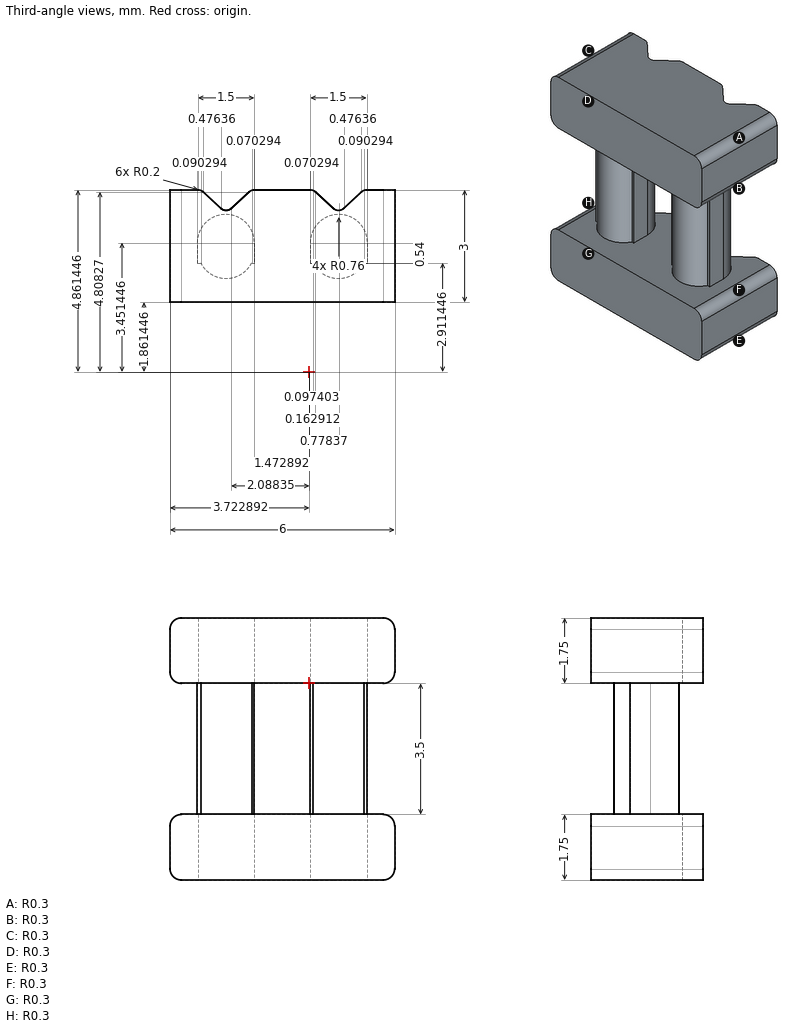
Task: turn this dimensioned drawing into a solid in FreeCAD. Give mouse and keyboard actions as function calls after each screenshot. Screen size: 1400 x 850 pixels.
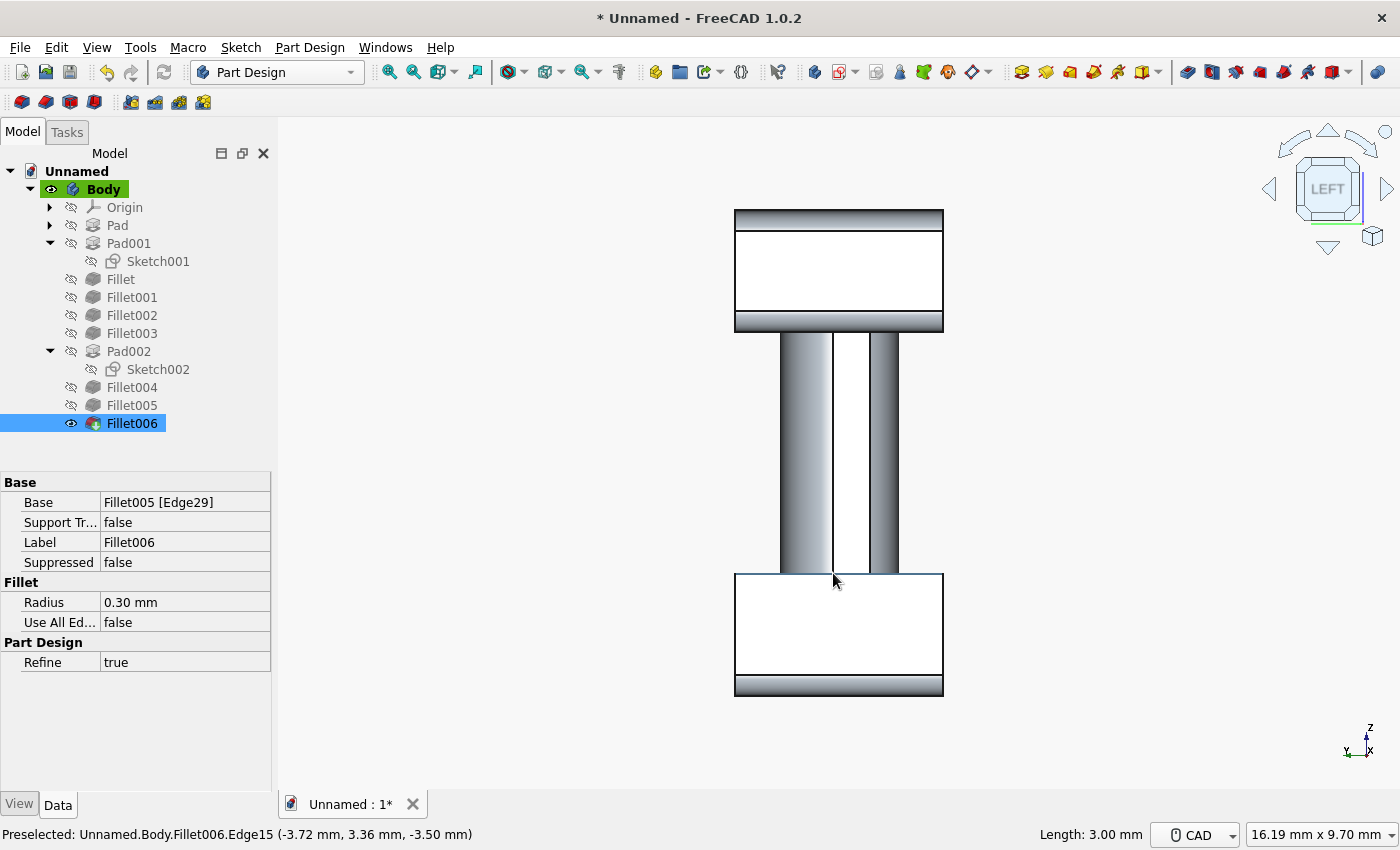
click(22, 102)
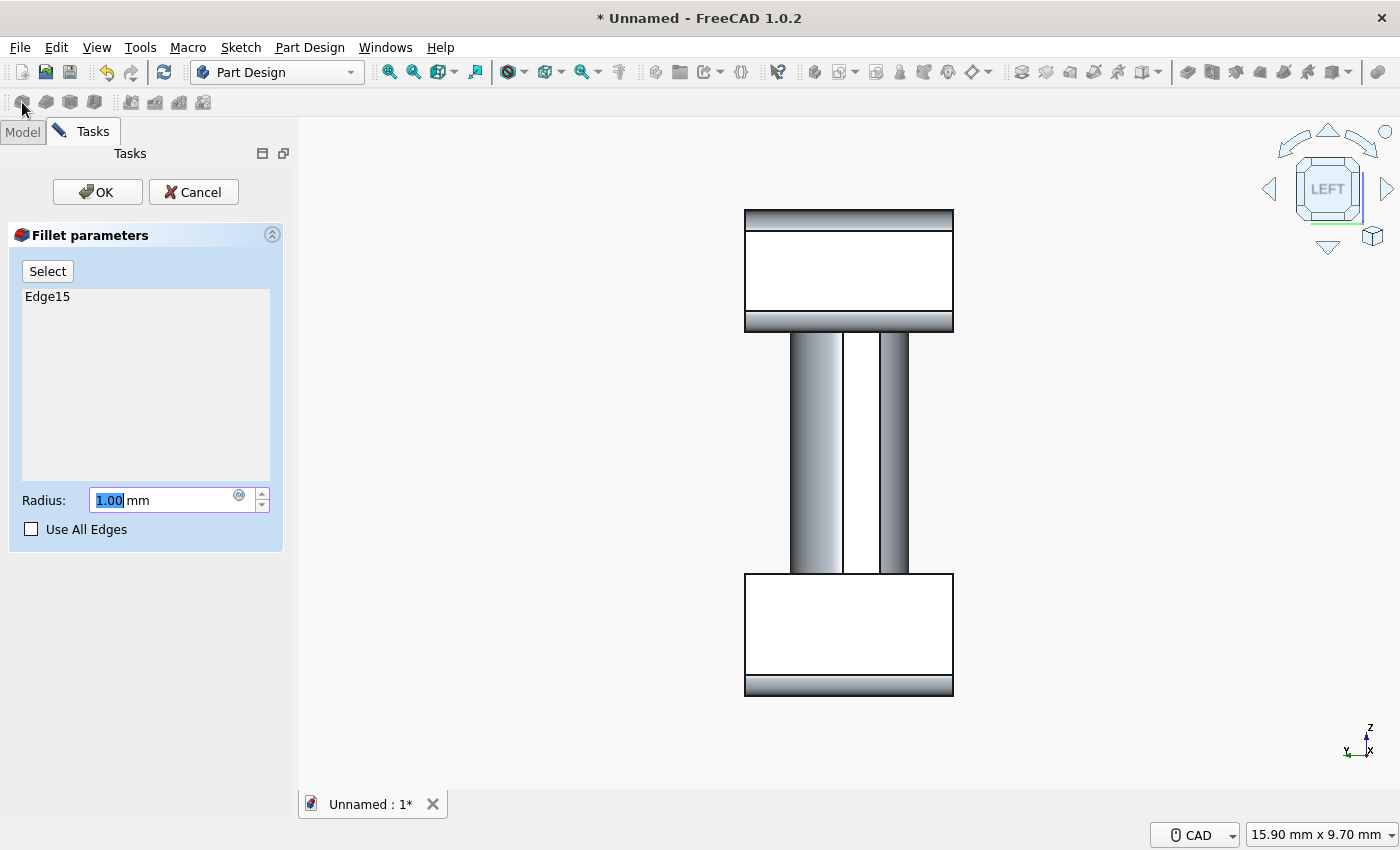
text(0.3)
key(Tab)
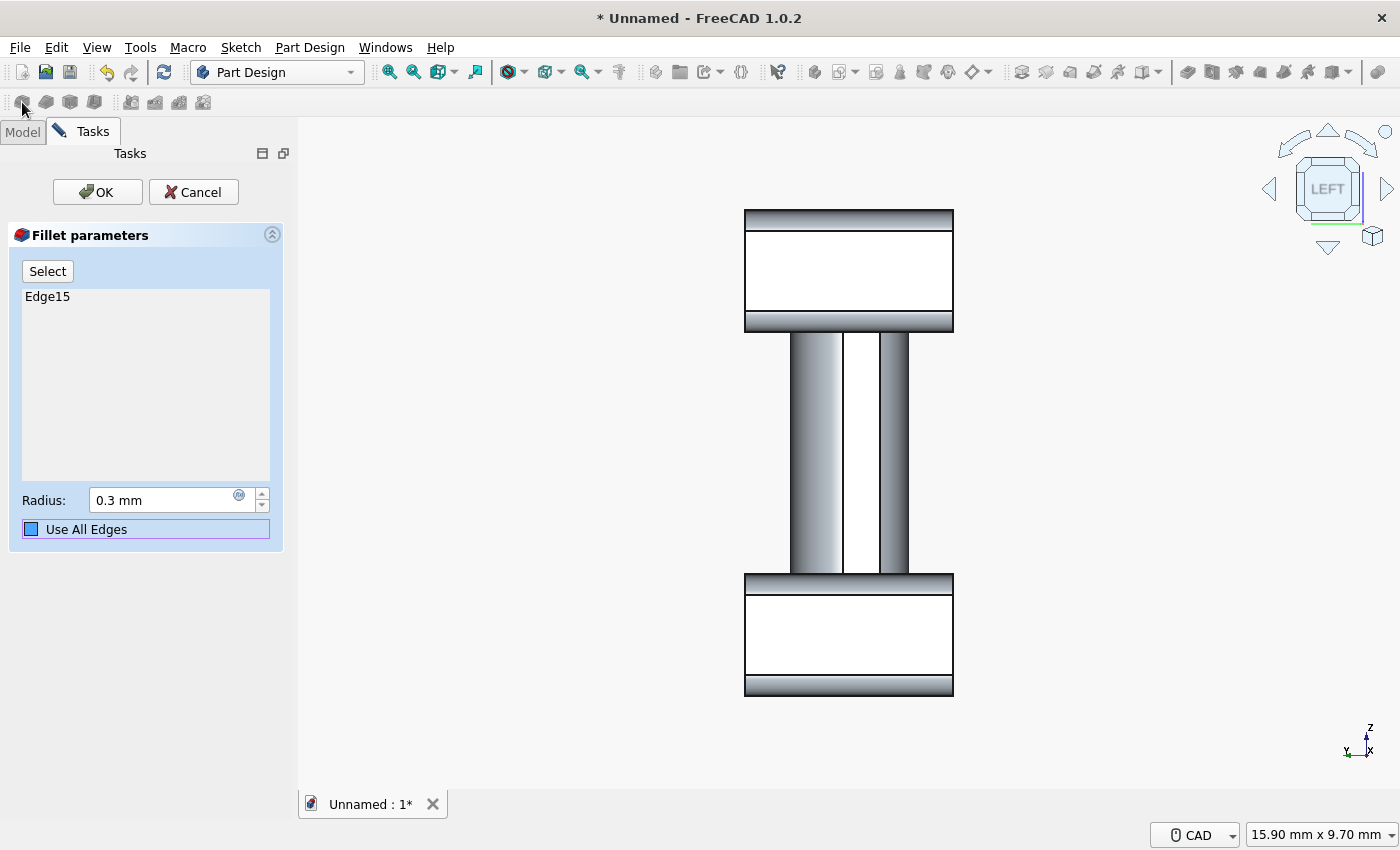
click(98, 192)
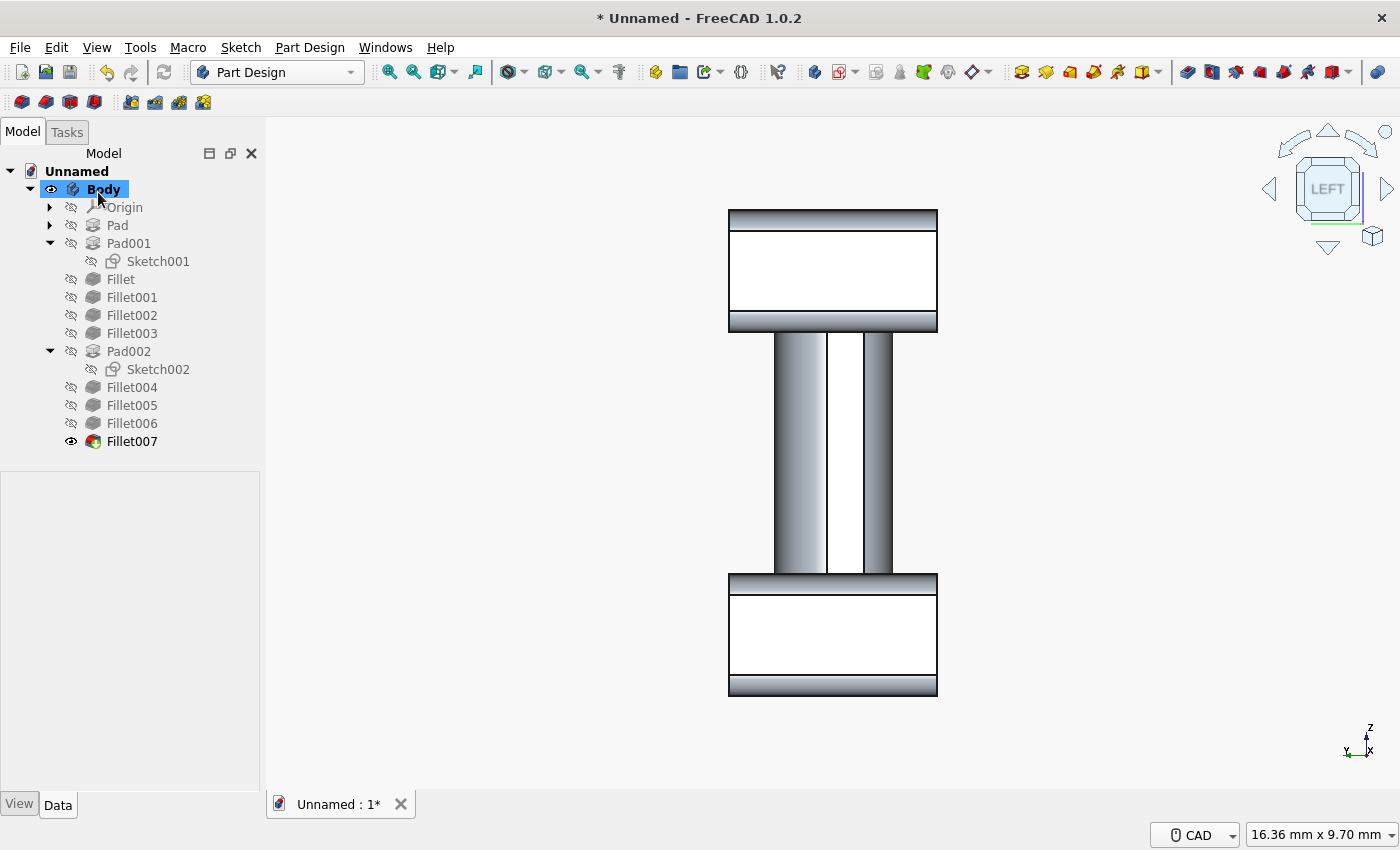
key(0)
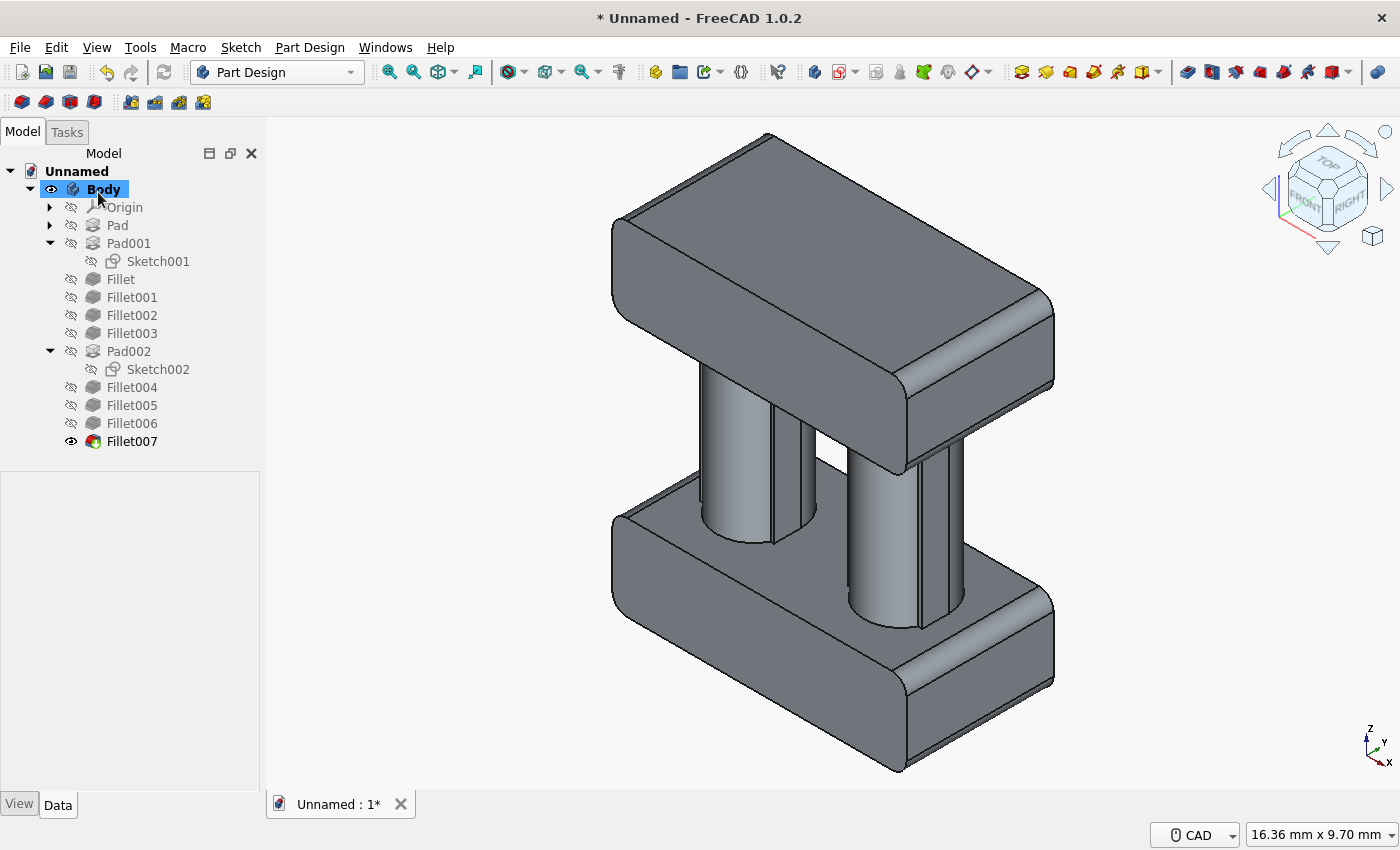
click(871, 276)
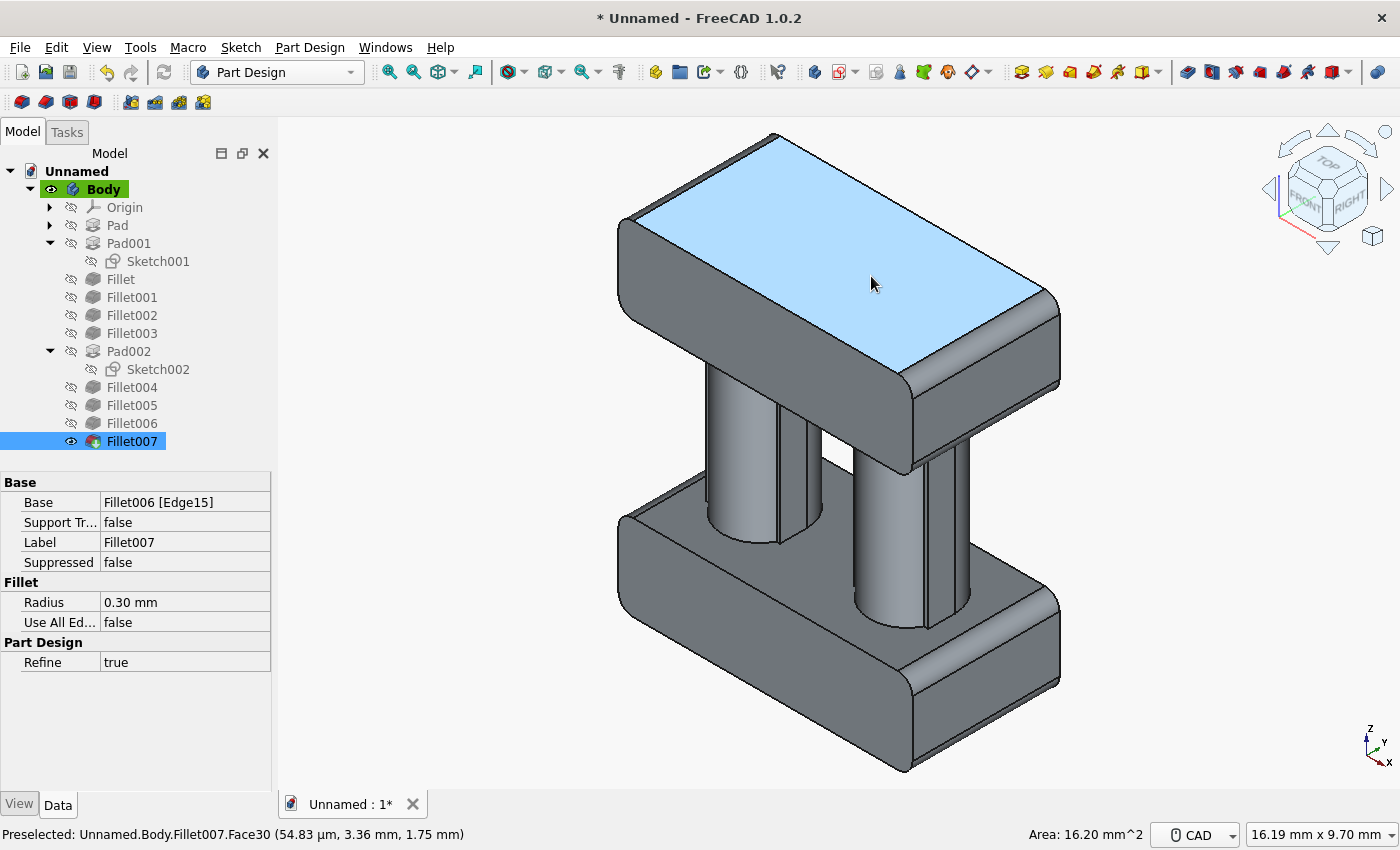
click(840, 72)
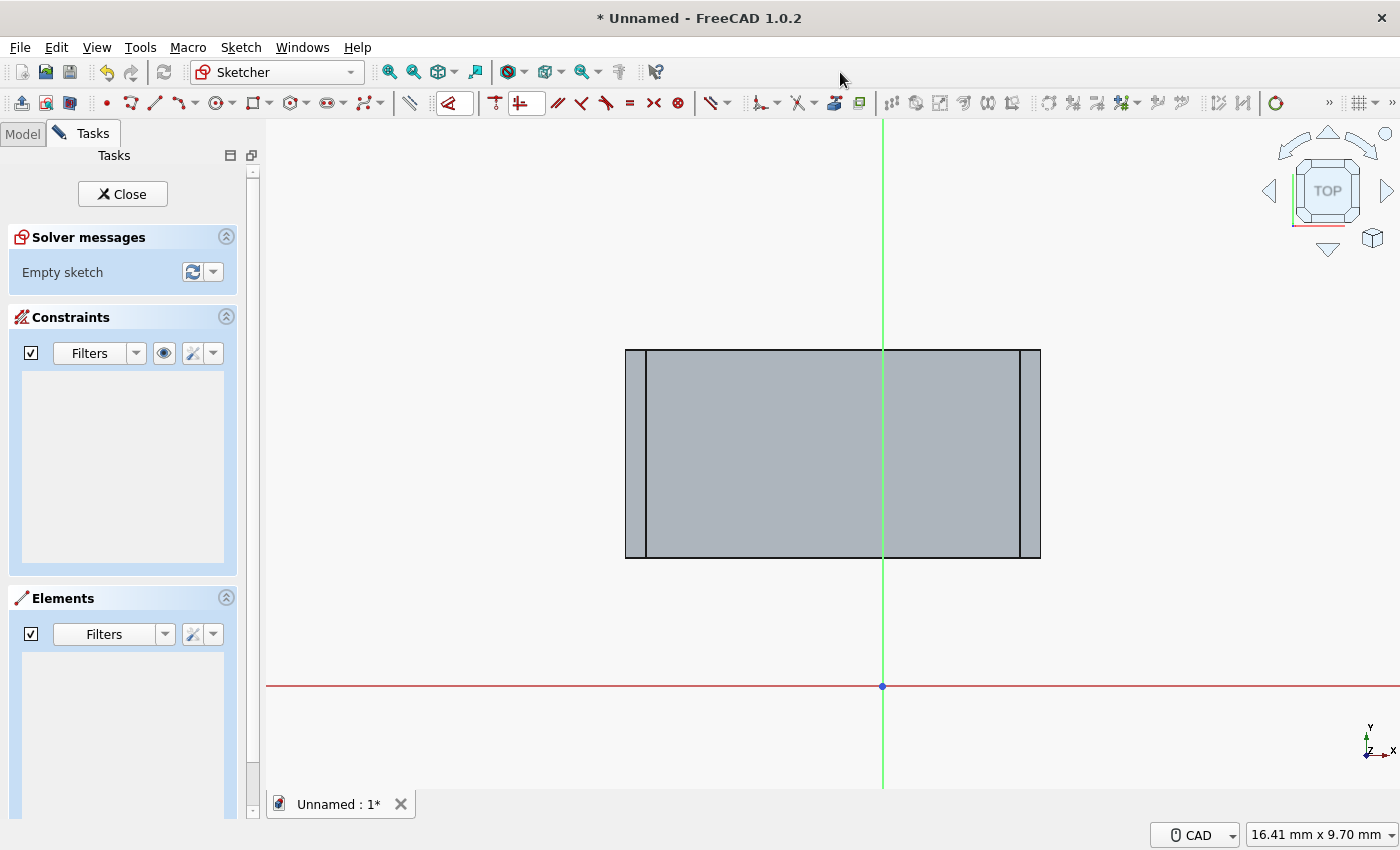
click(156, 104)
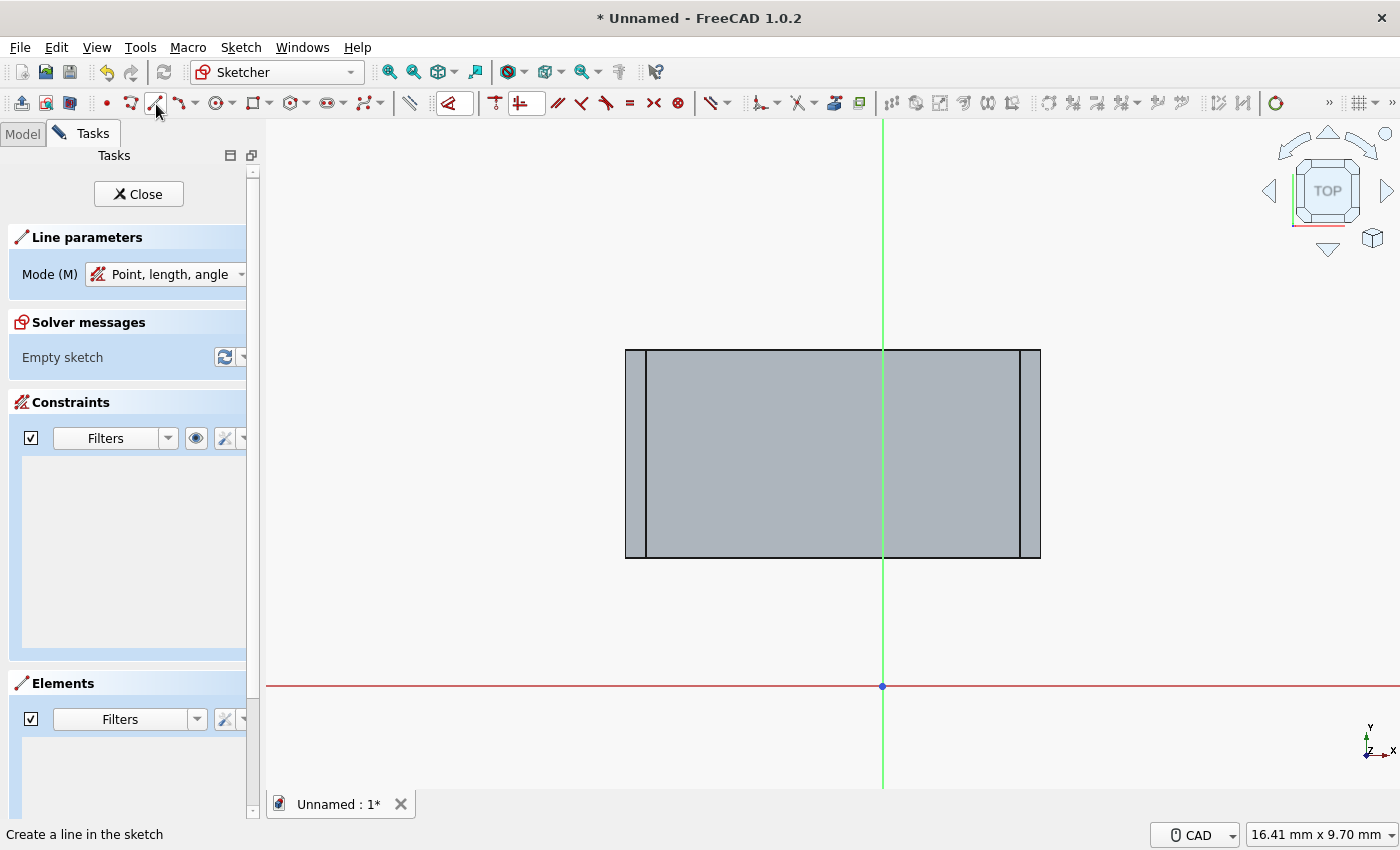
click(781, 350)
click(678, 350)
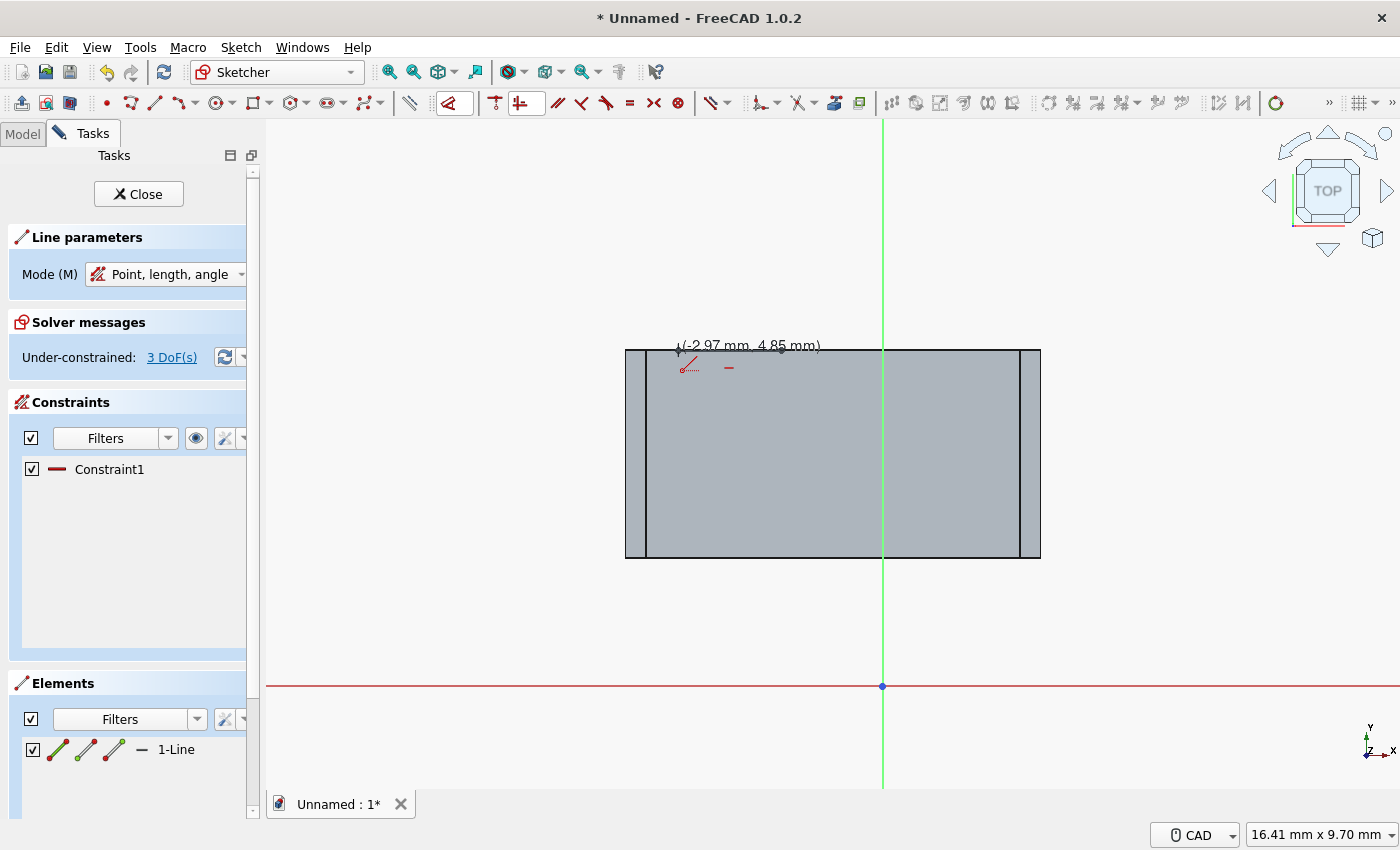
scroll(687, 354, up, 8)